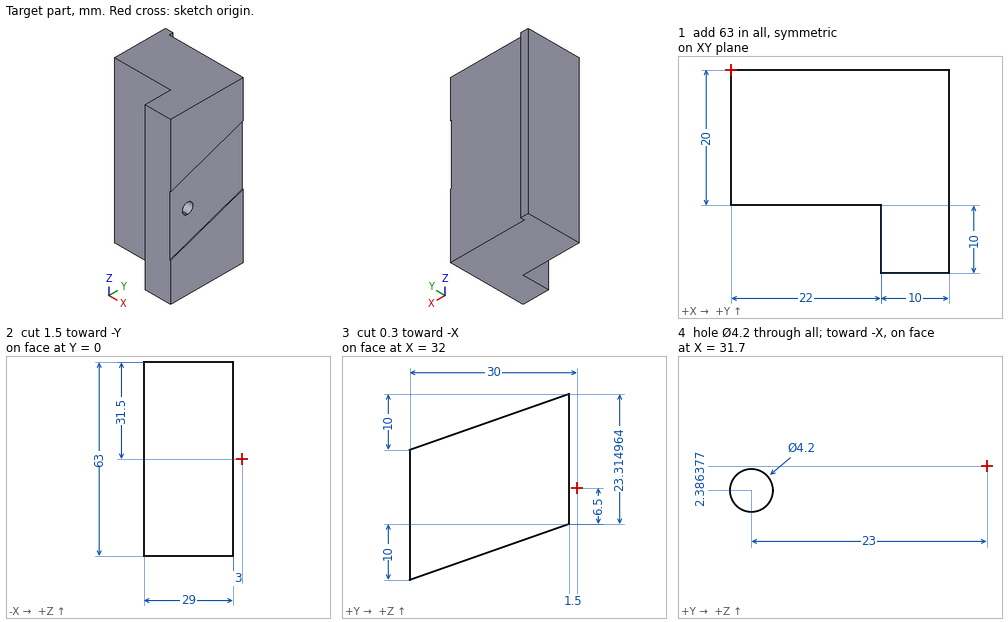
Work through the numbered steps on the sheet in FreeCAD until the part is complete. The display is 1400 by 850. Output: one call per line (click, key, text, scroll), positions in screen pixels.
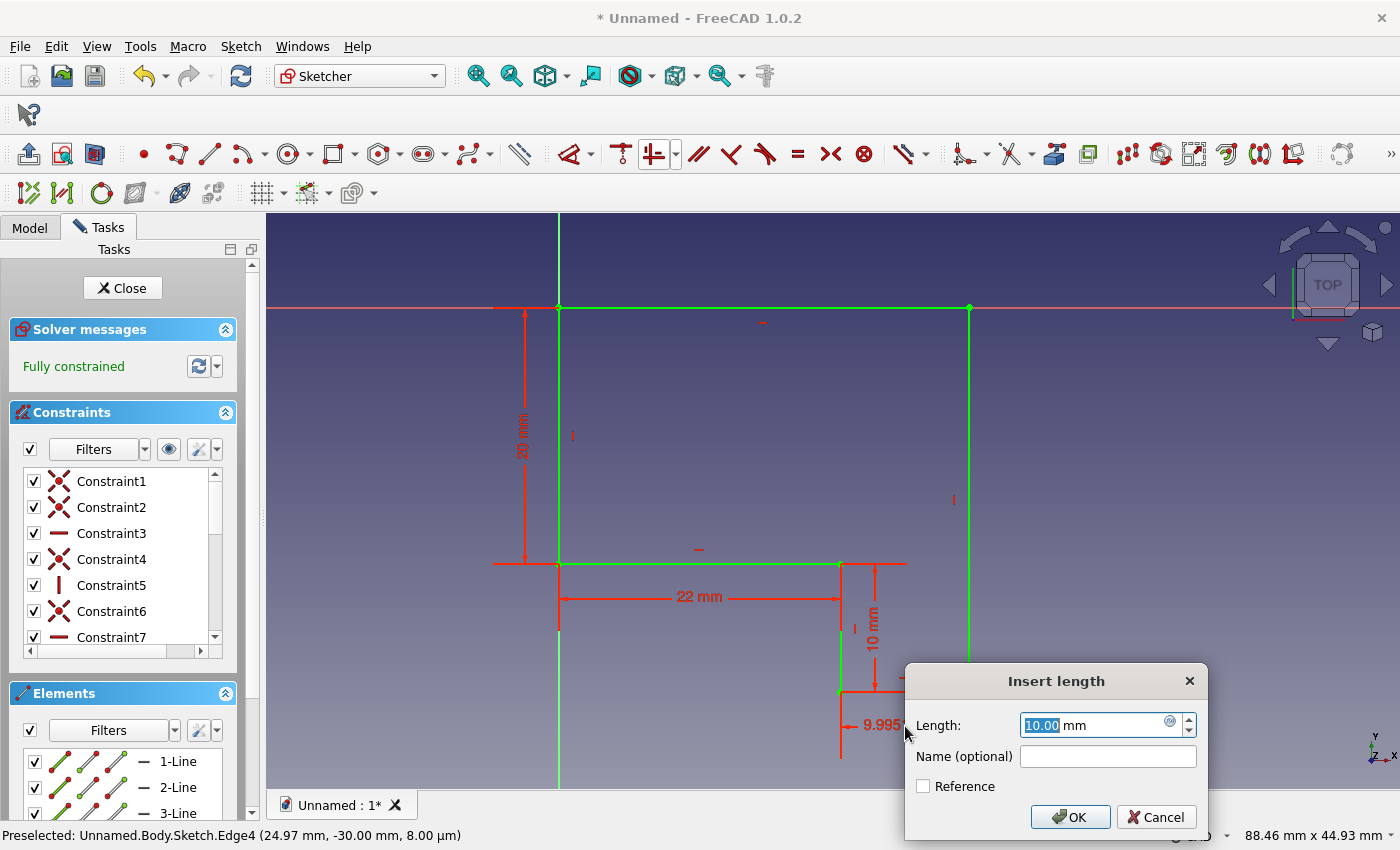
text(10)
key(Return)
key(Escape)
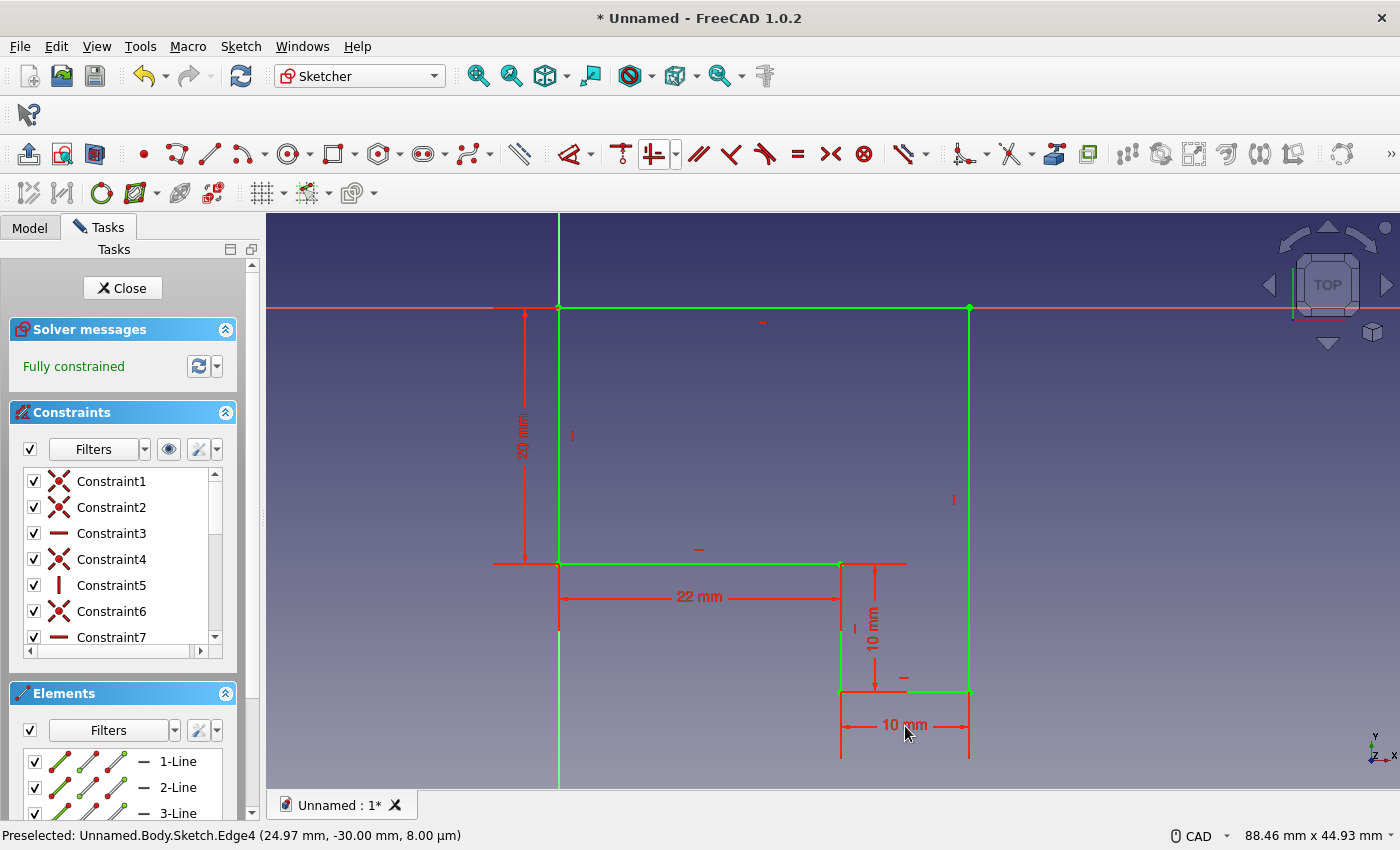
click(123, 288)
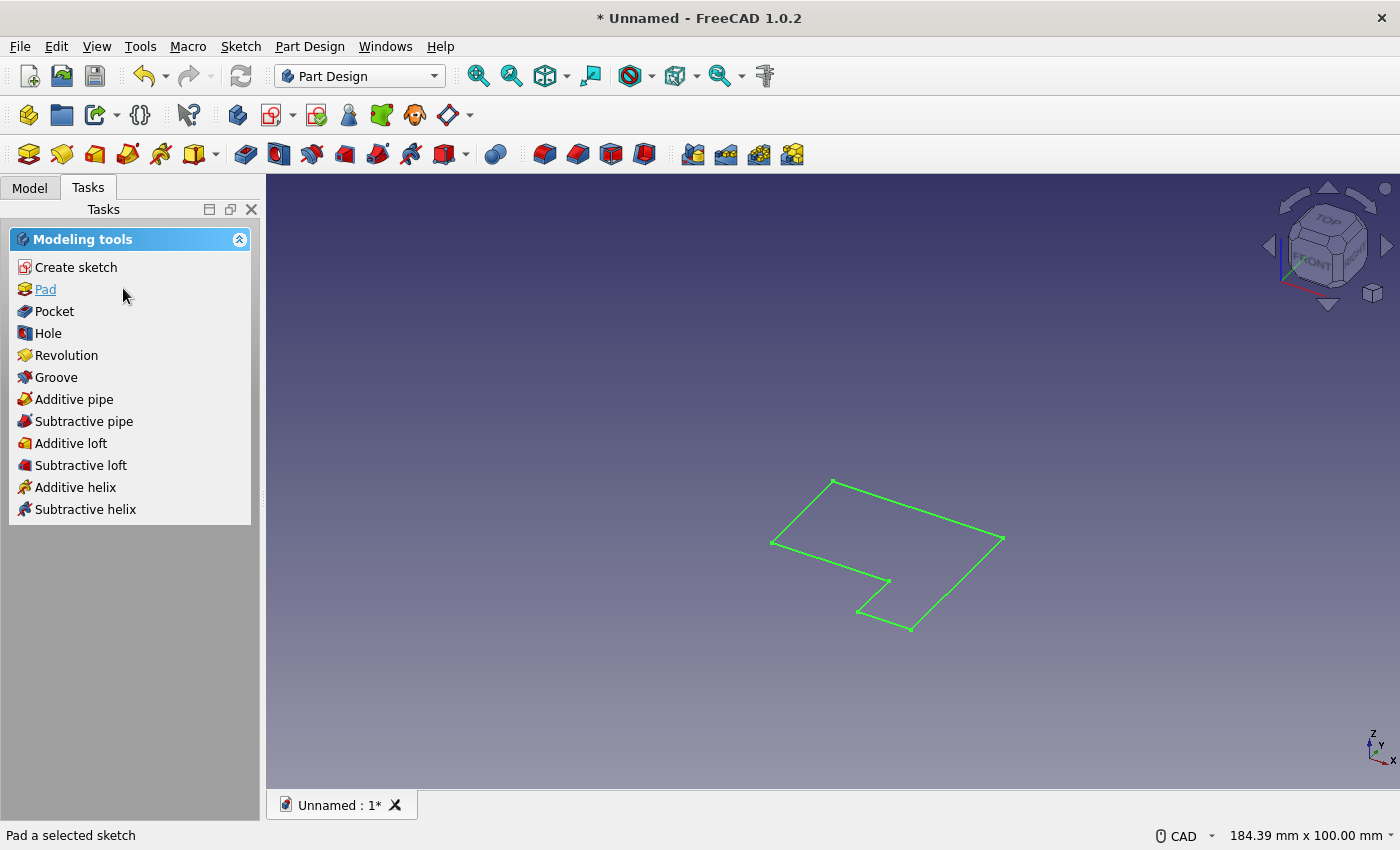
click(29, 154)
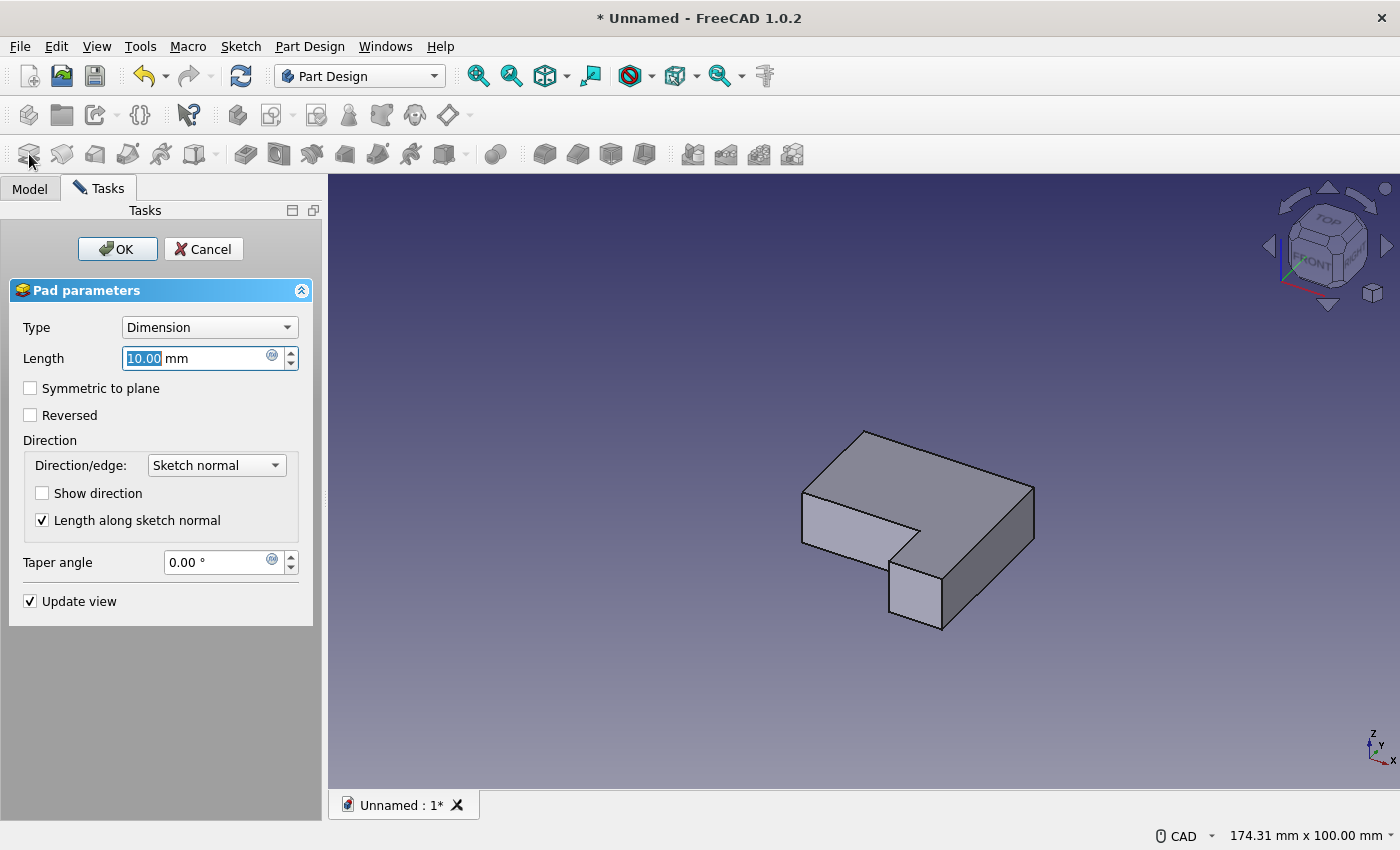
text(63)
key(Tab)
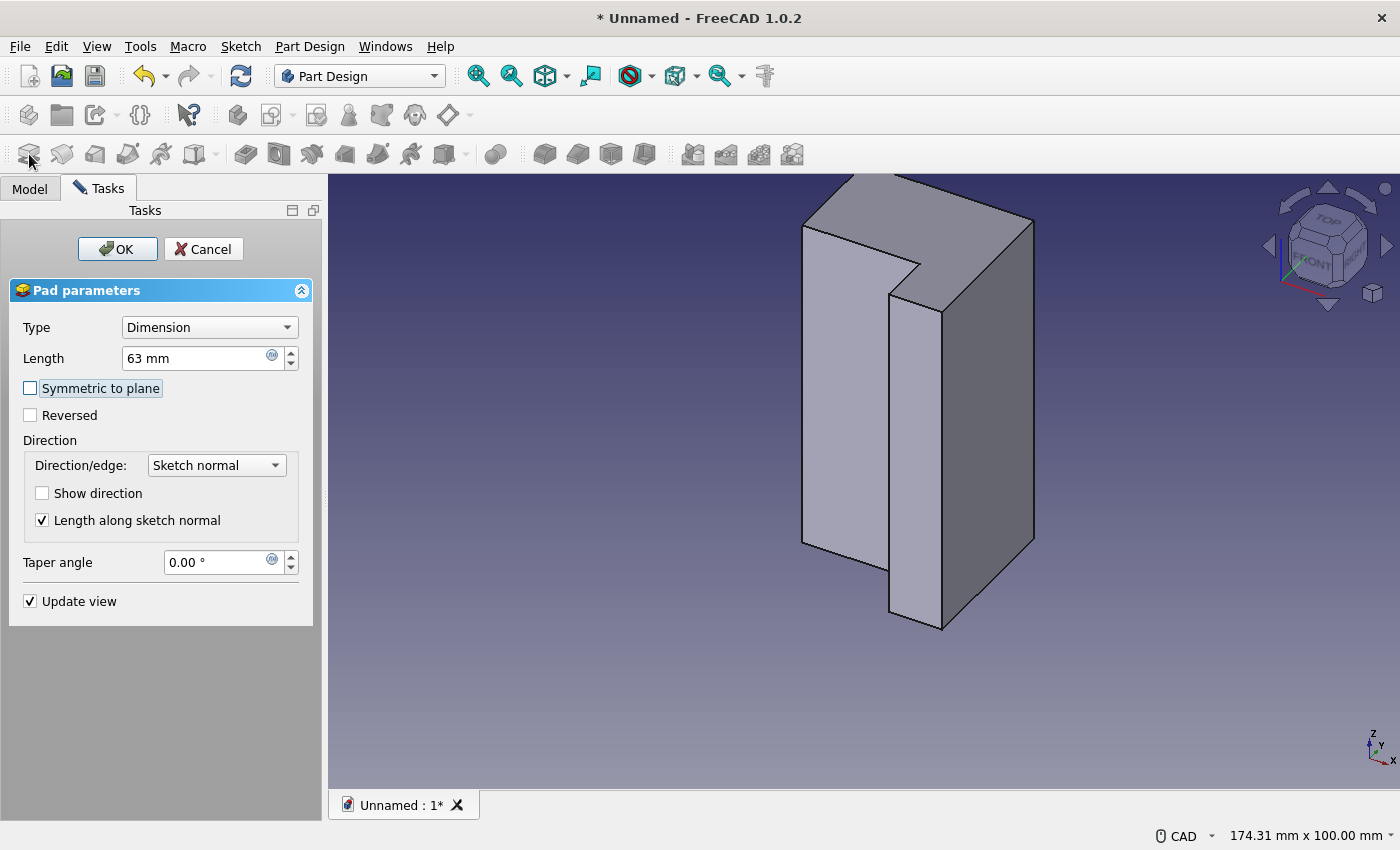
click(31, 388)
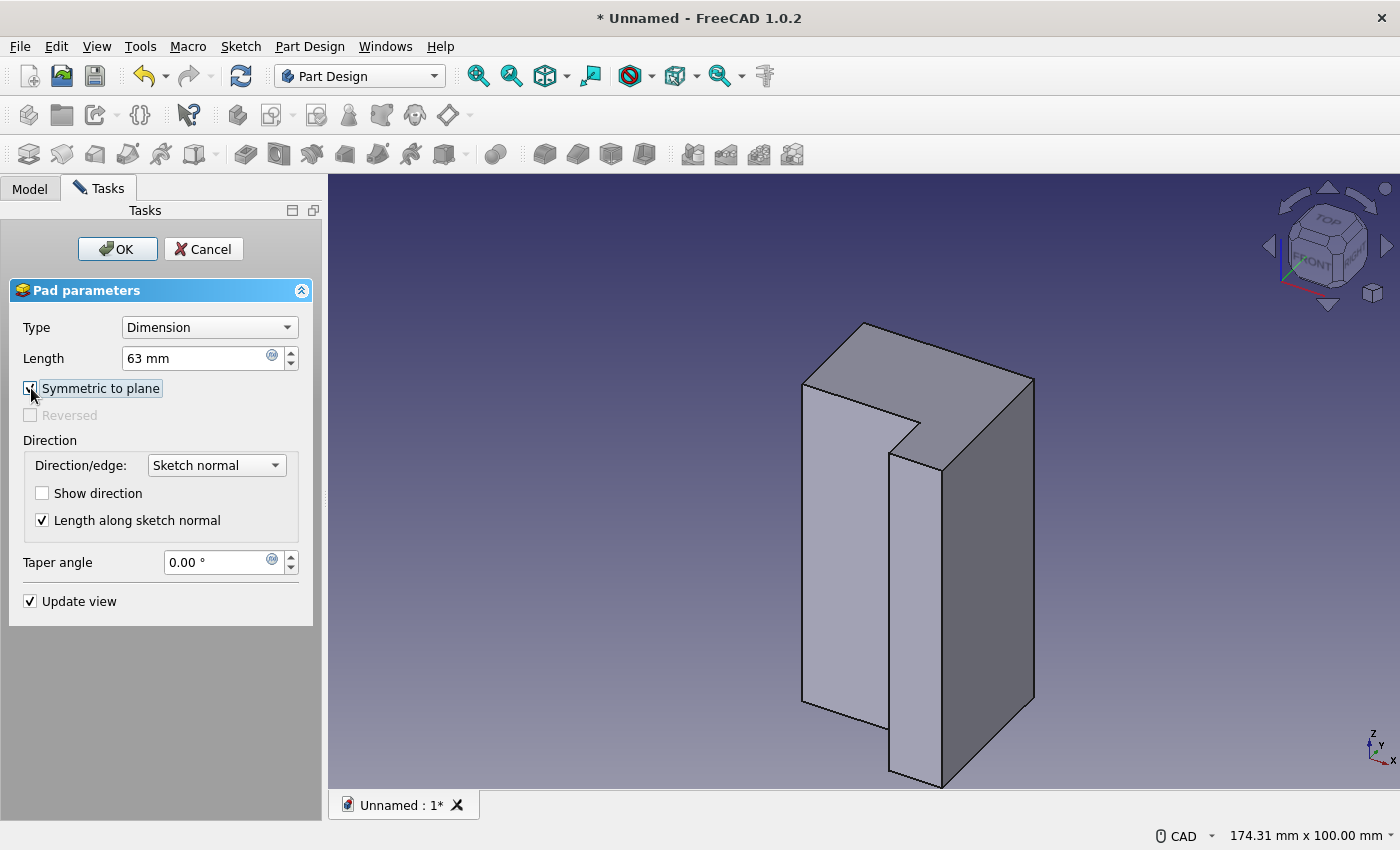
click(118, 249)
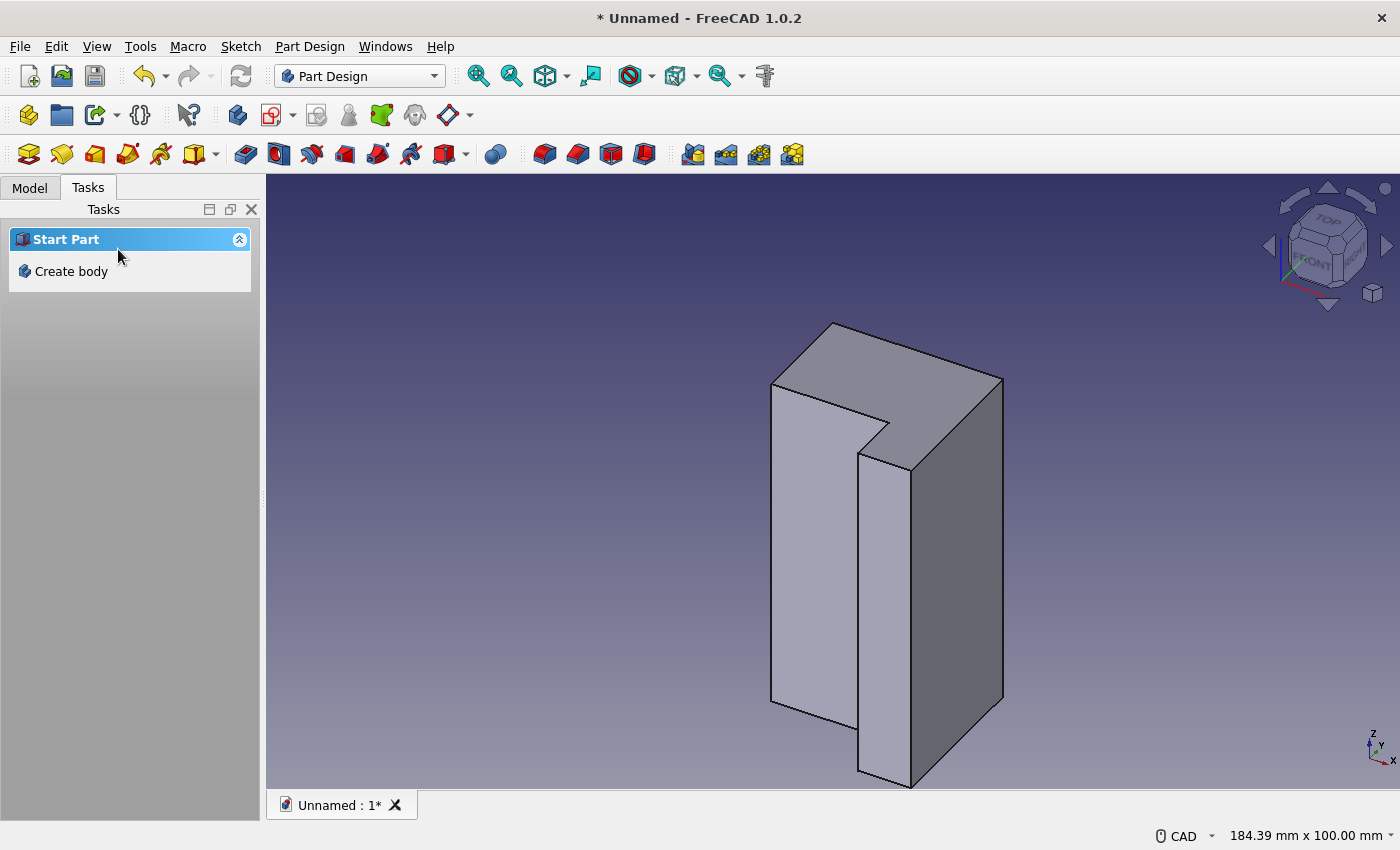
key(4)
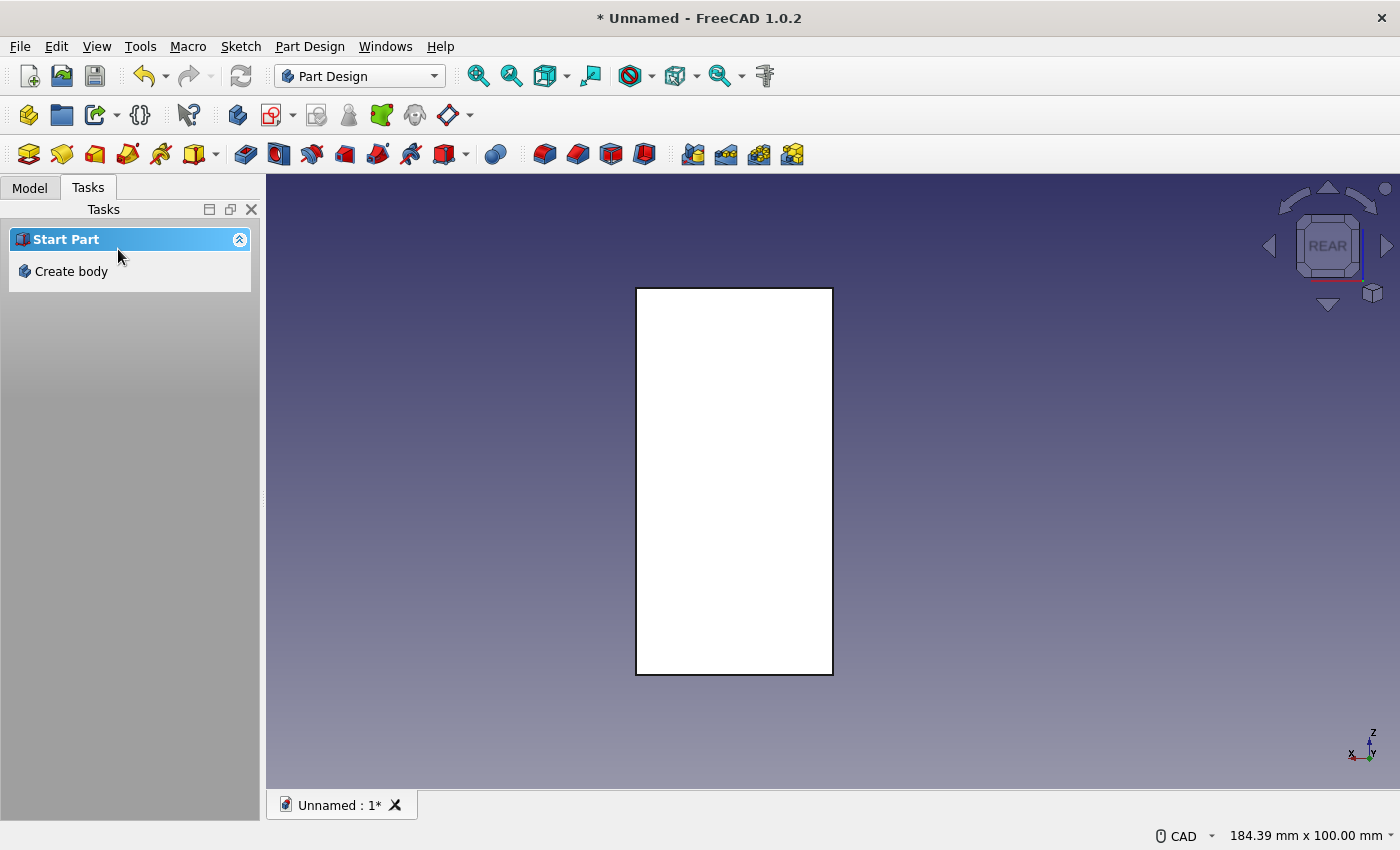
click(735, 425)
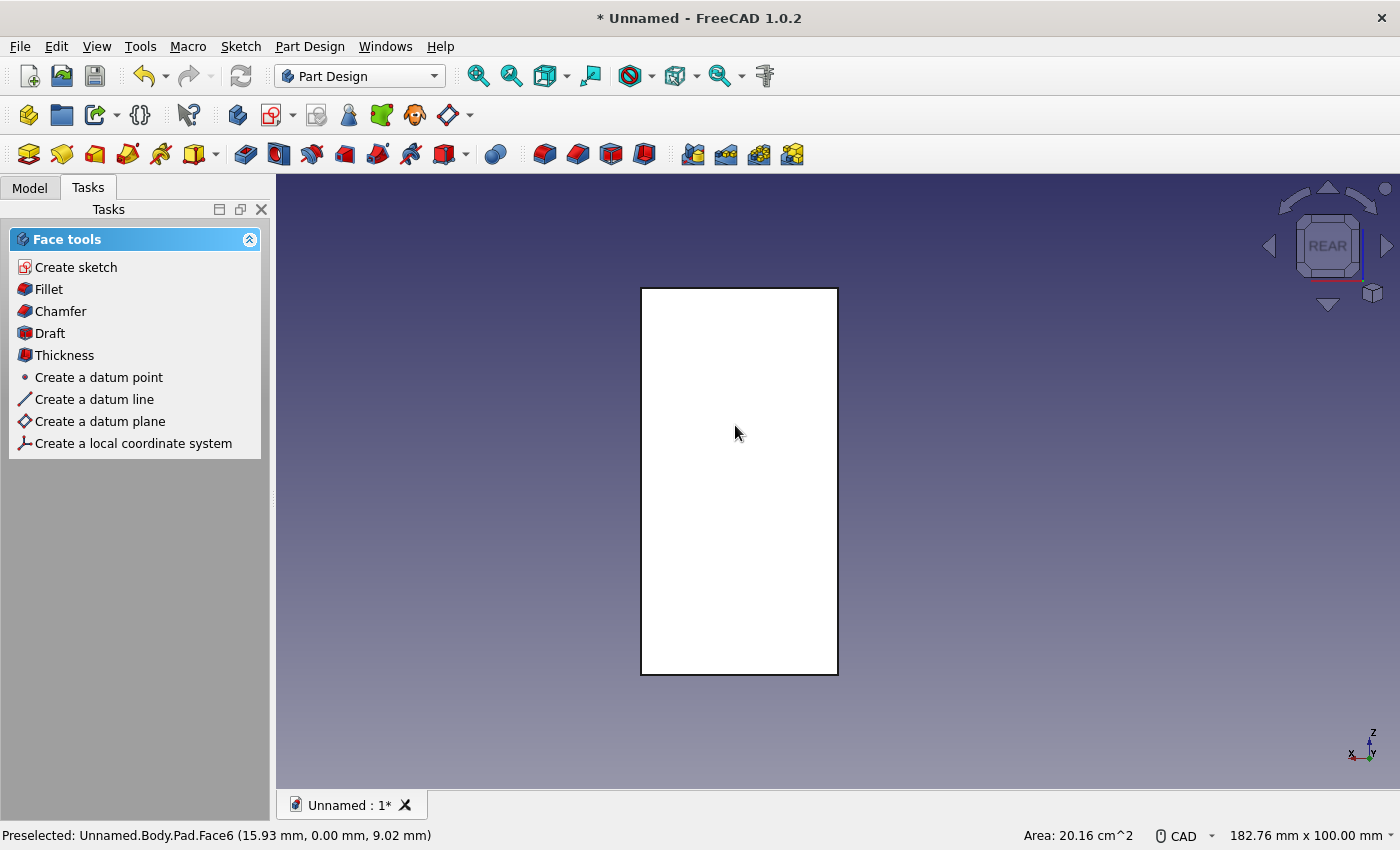
click(270, 116)